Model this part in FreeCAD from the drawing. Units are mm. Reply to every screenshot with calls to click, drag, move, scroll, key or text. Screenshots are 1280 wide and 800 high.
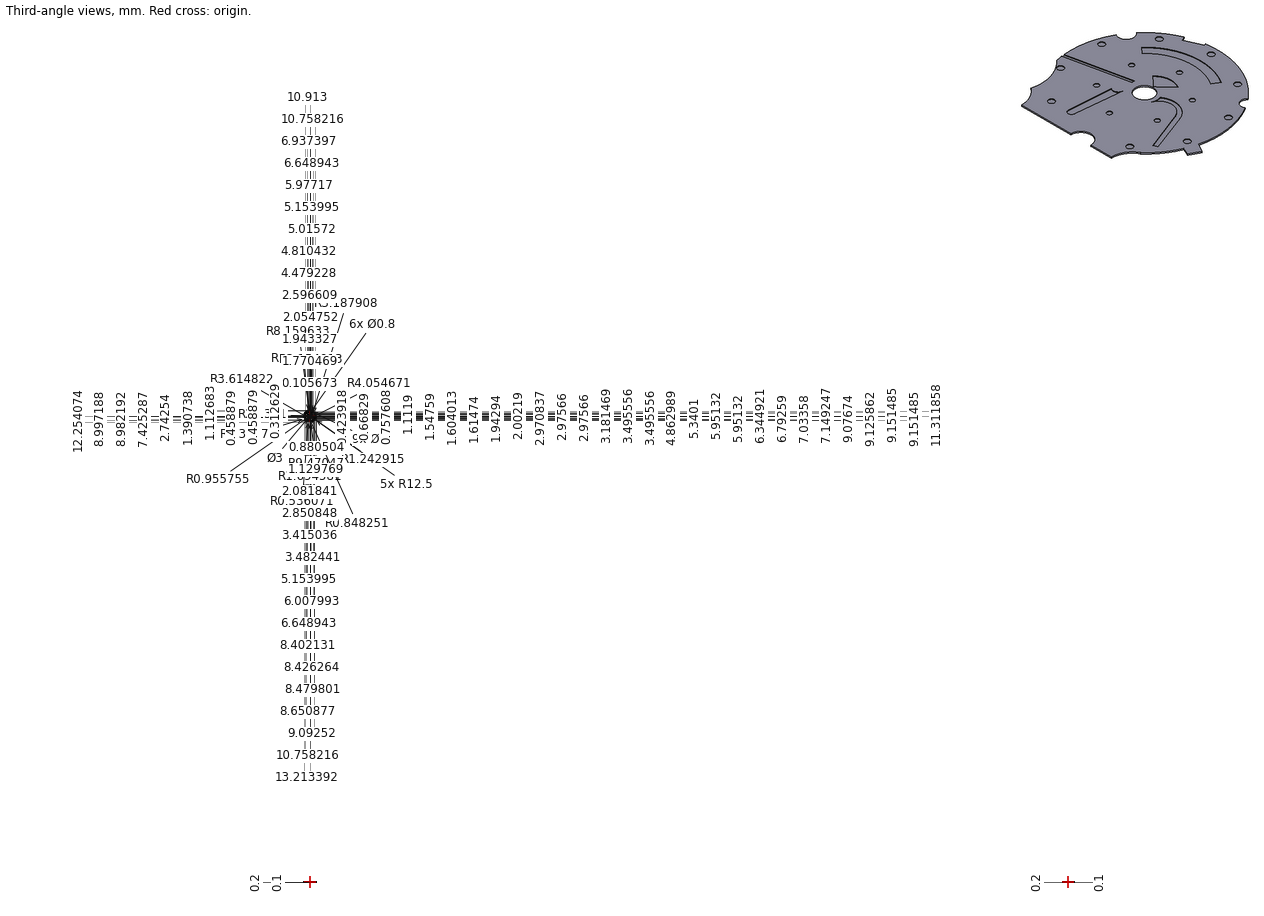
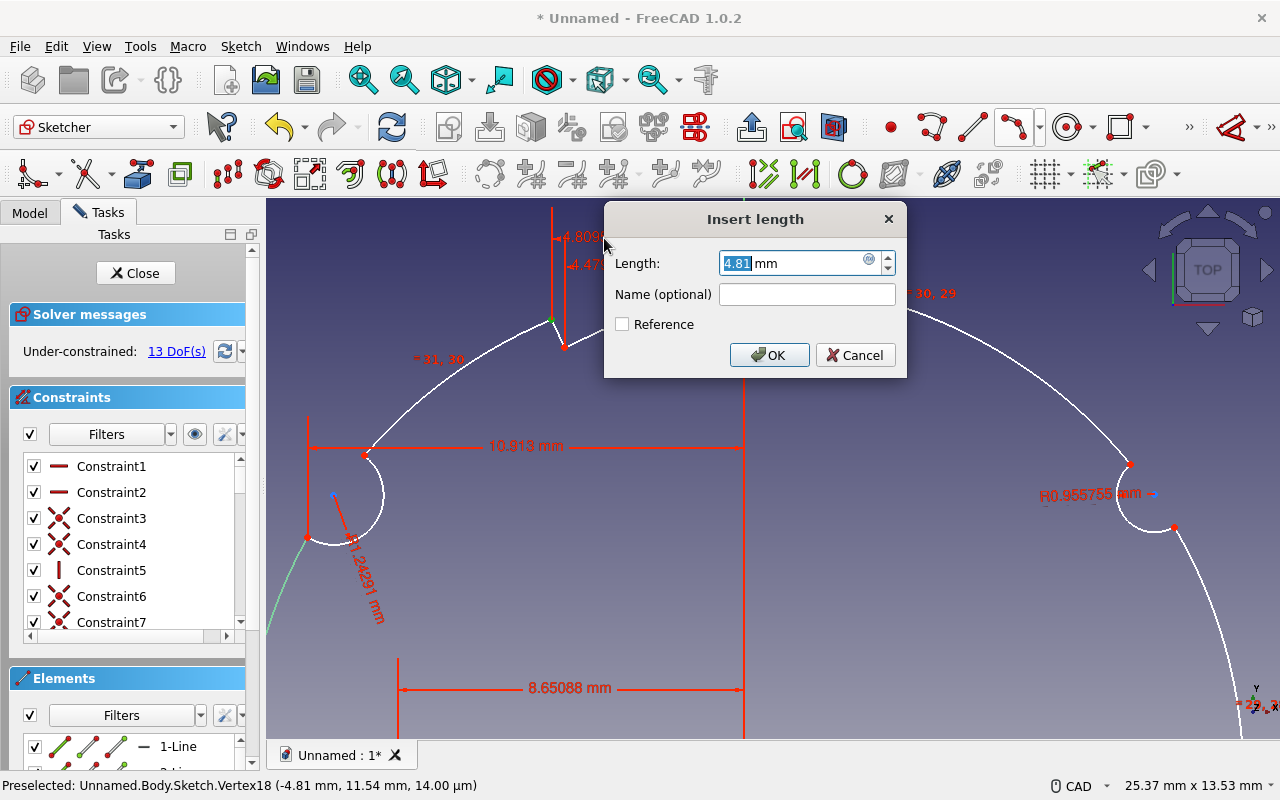
text(4.810432)
key(Return)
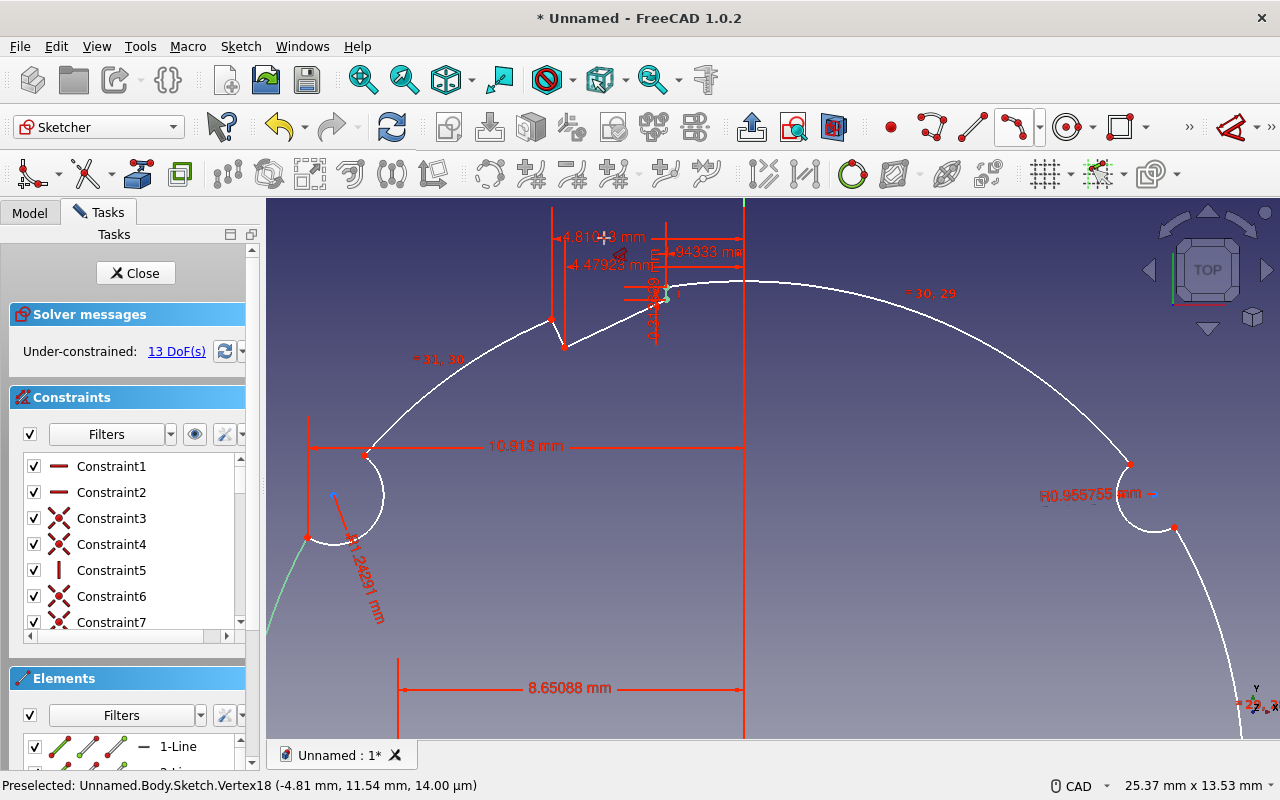
scroll(668, 288, down, 5)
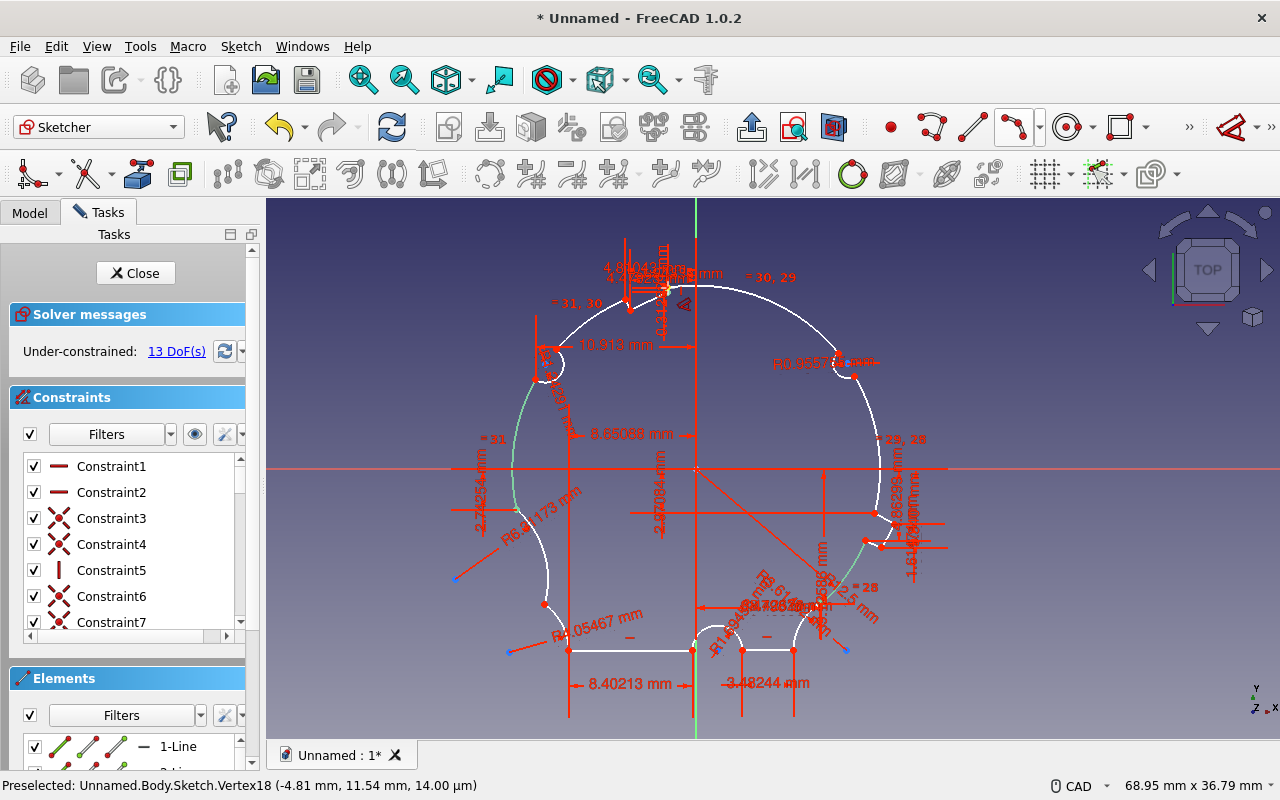
scroll(820, 604, up, 13)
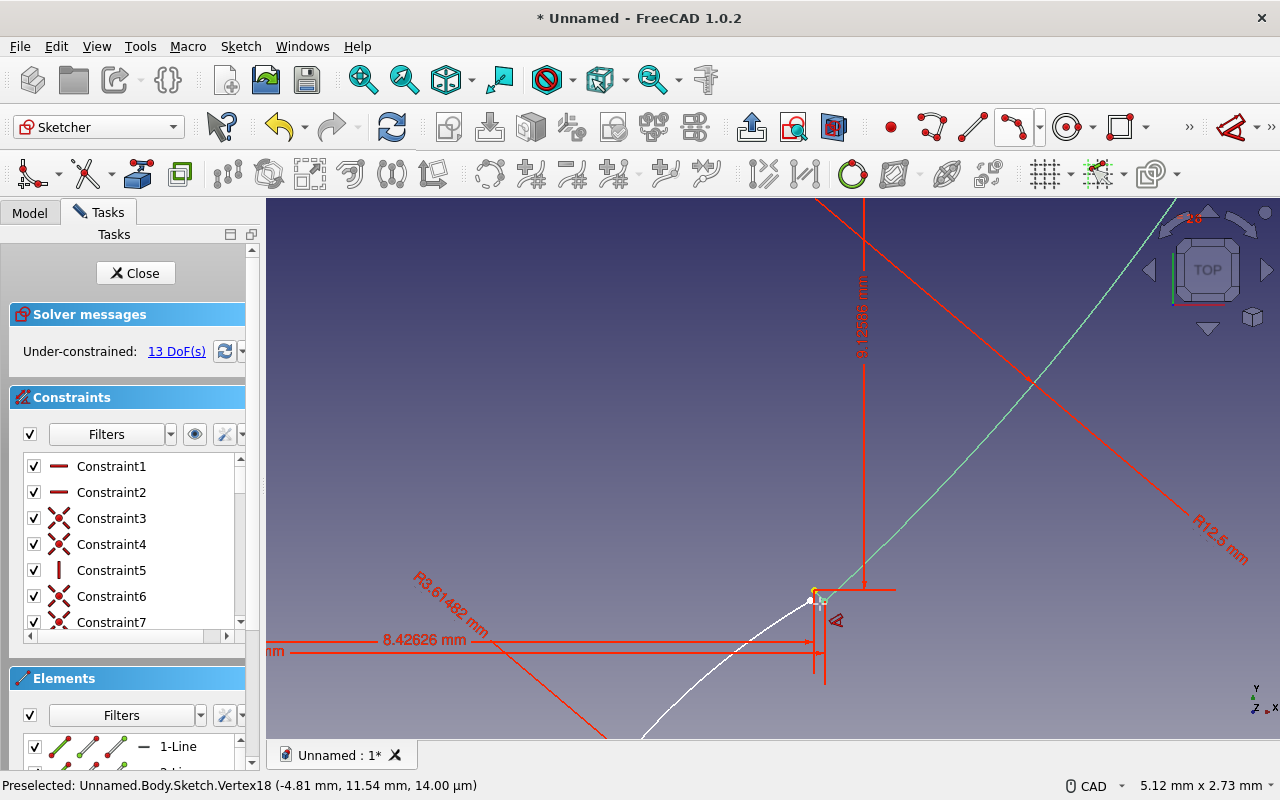
click(811, 601)
click(552, 635)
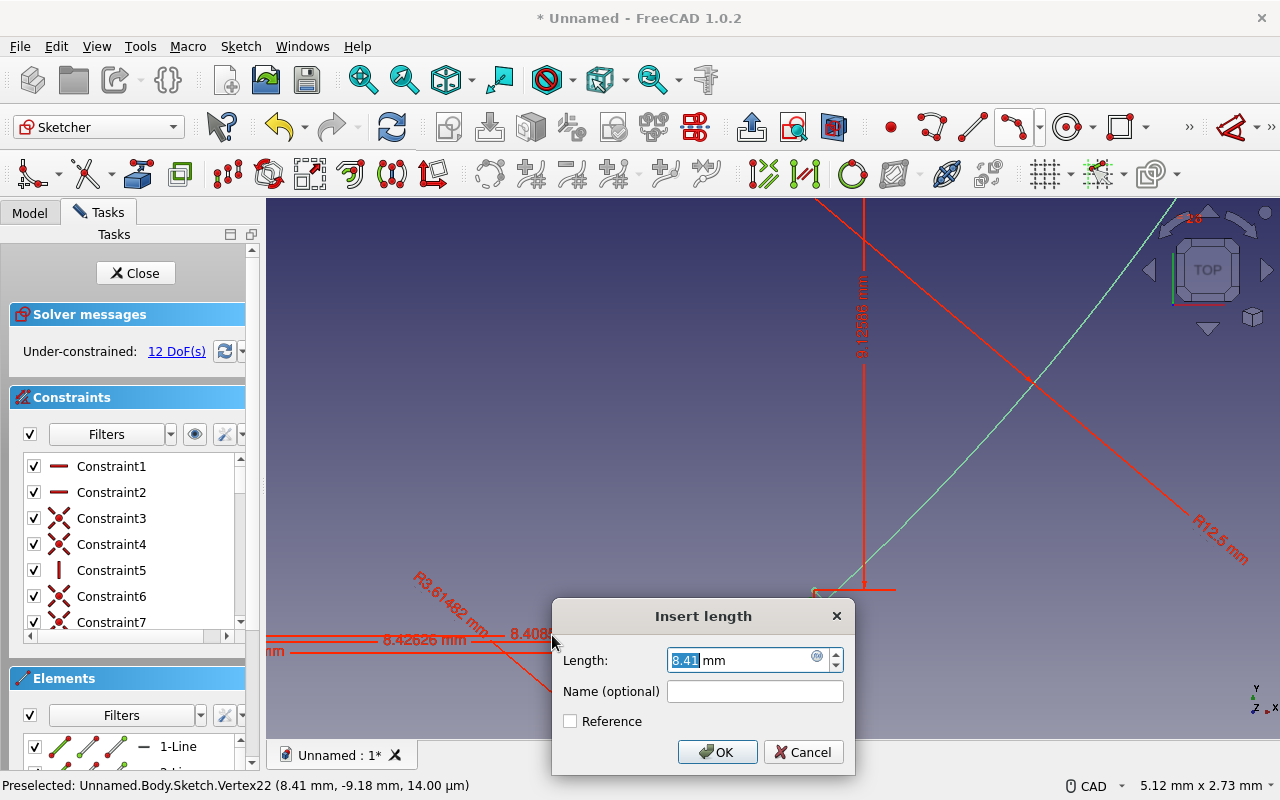
text(8.426264)
key(Return)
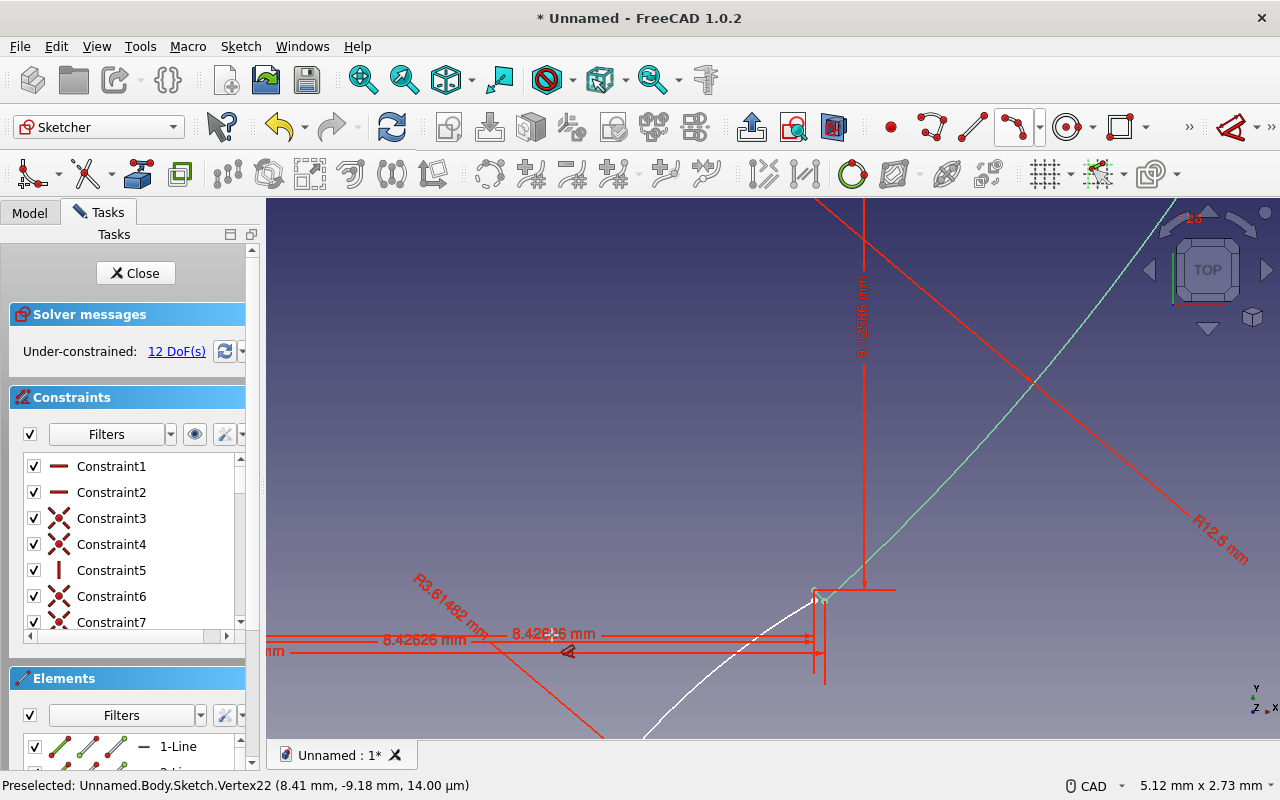
click(814, 601)
click(848, 413)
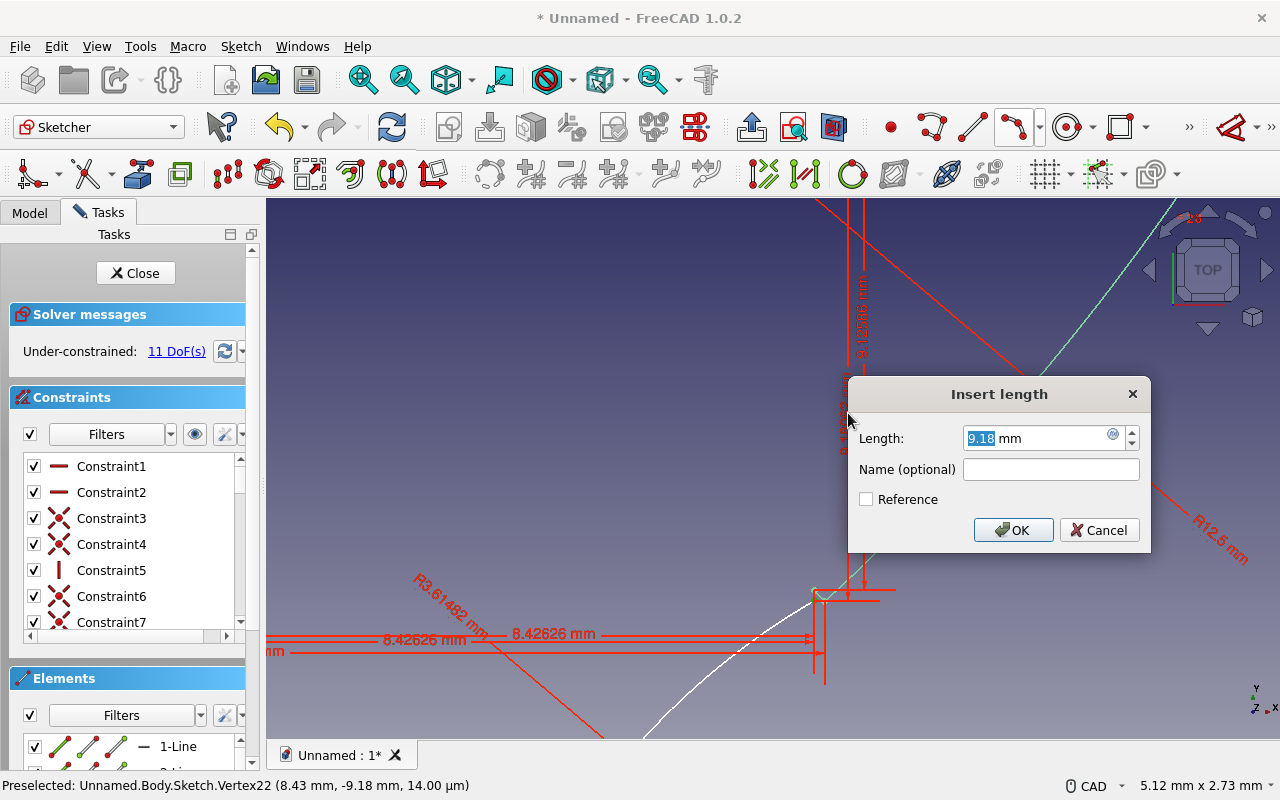
text(9.125862)
key(Return)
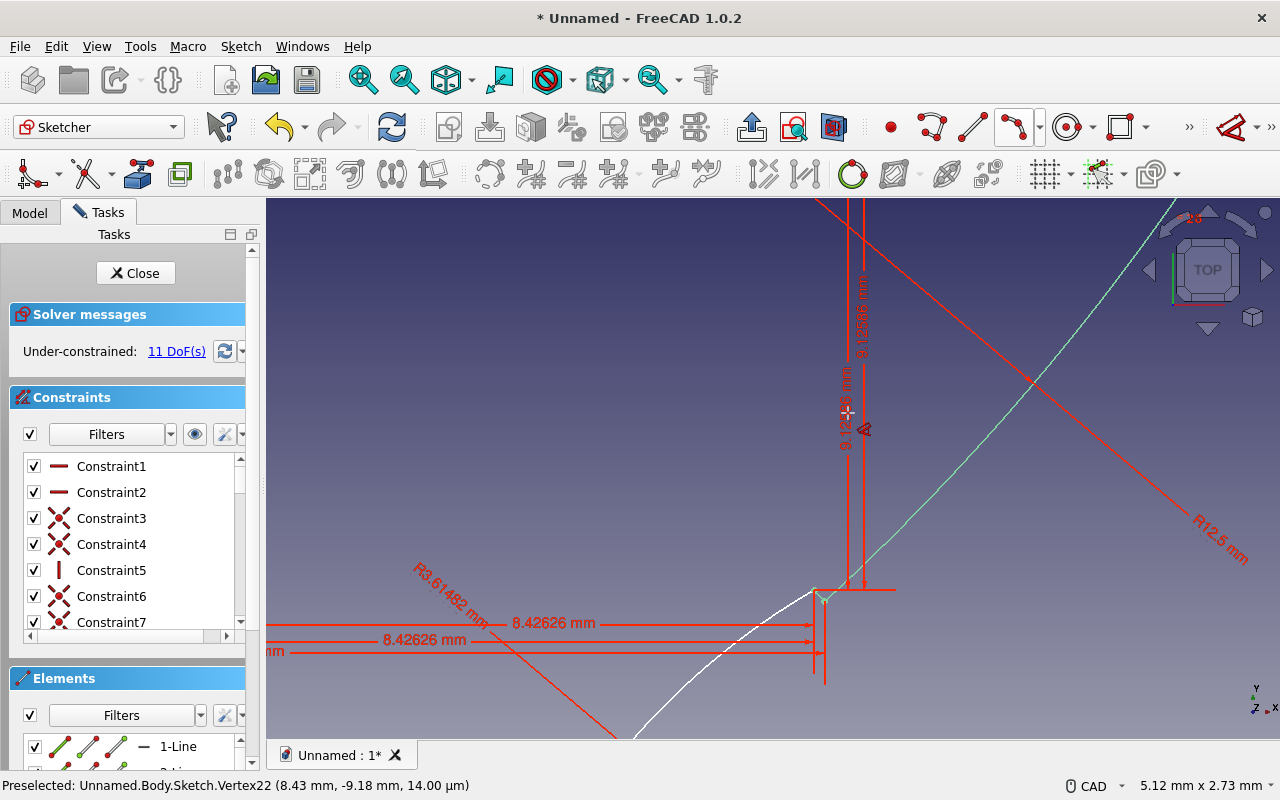
scroll(820, 604, down, 13)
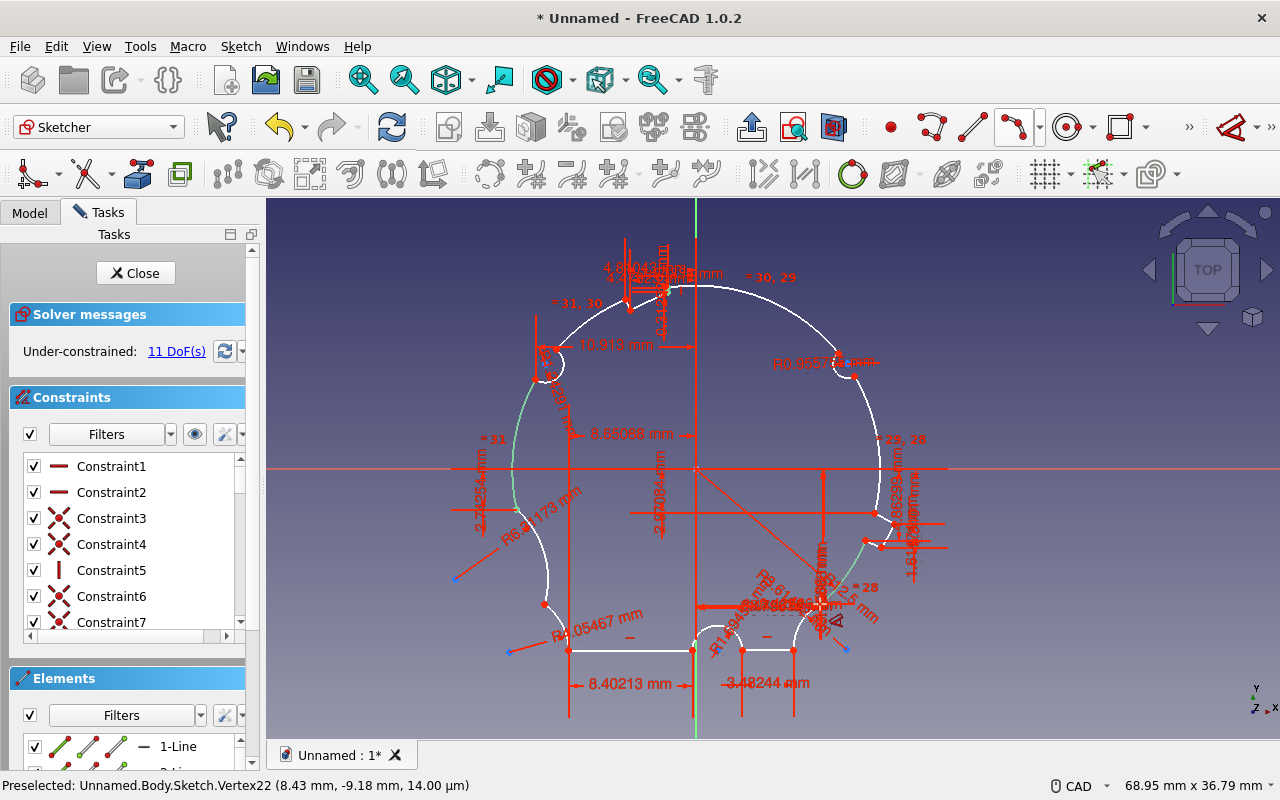
click(854, 376)
click(888, 423)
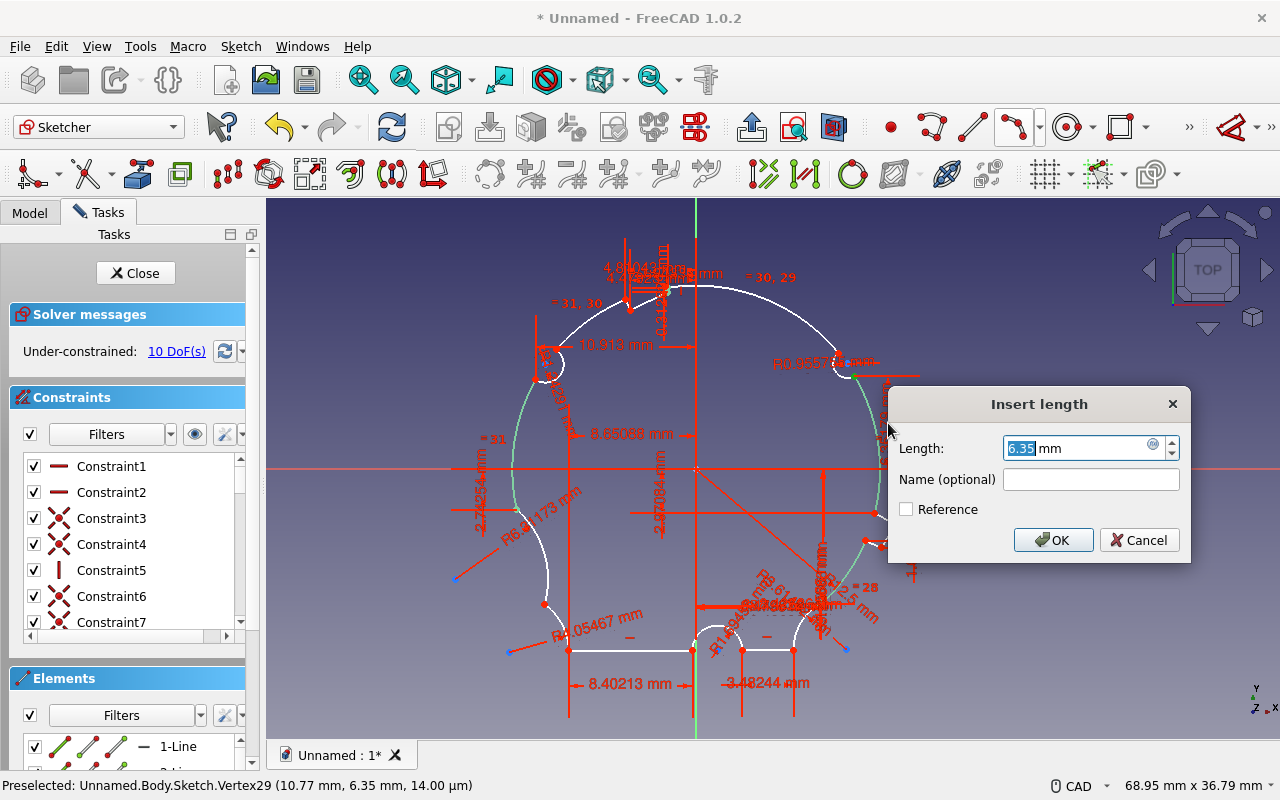
text(6.344921)
key(Return)